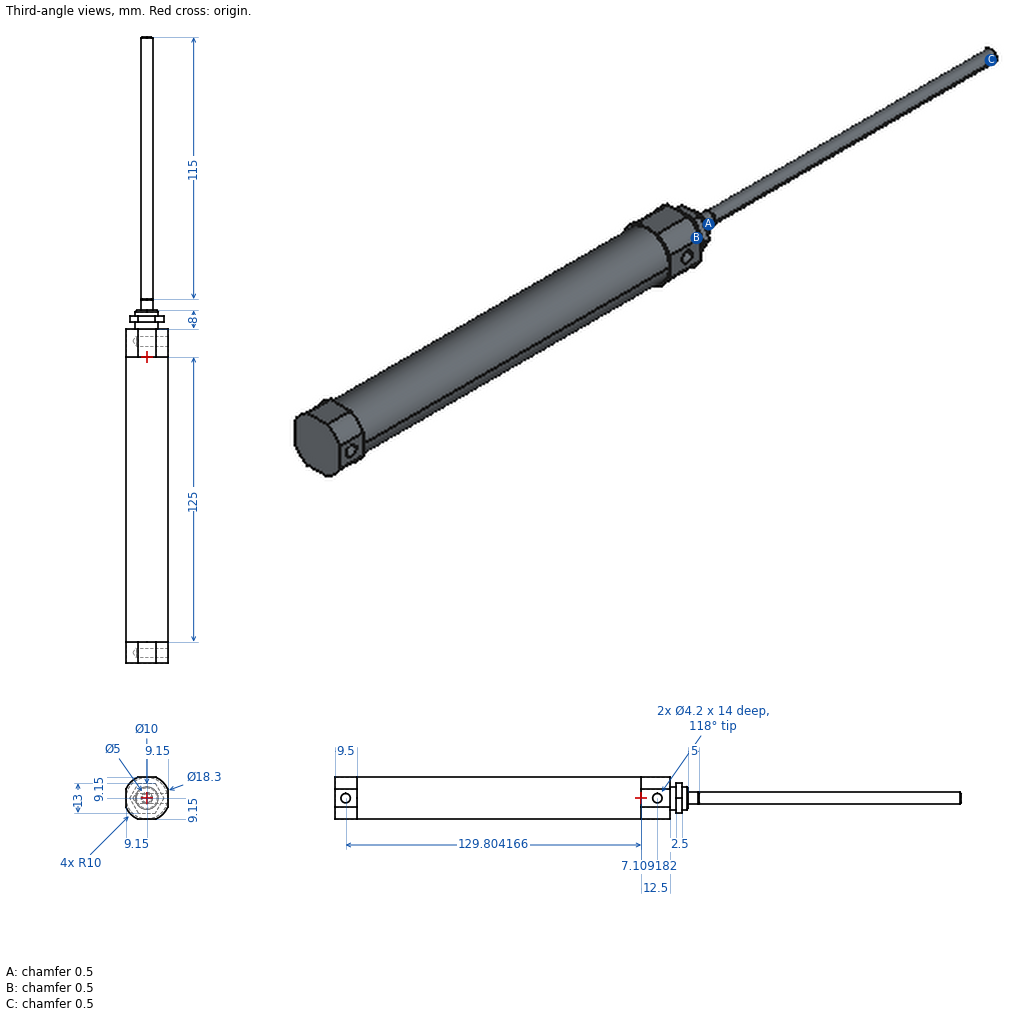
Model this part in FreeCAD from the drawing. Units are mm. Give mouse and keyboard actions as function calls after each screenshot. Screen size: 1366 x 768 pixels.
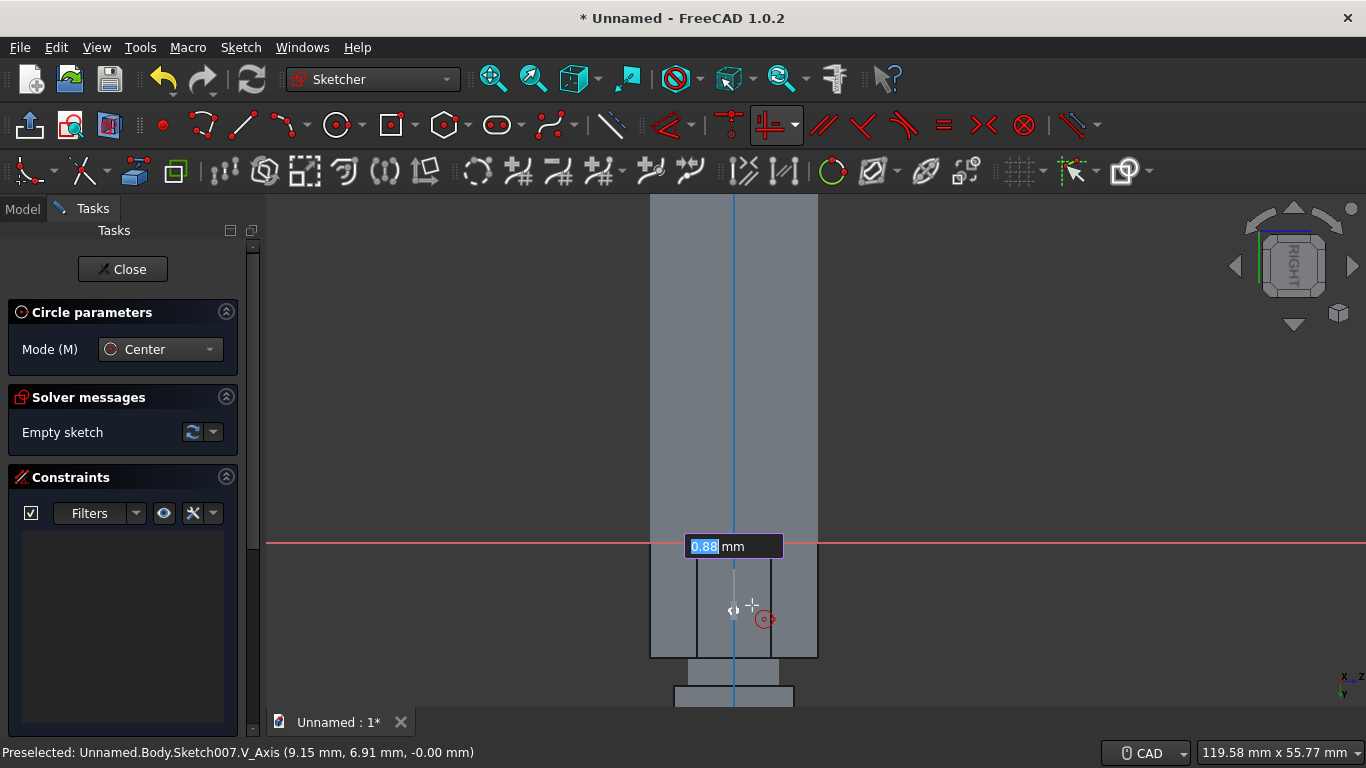
click(752, 602)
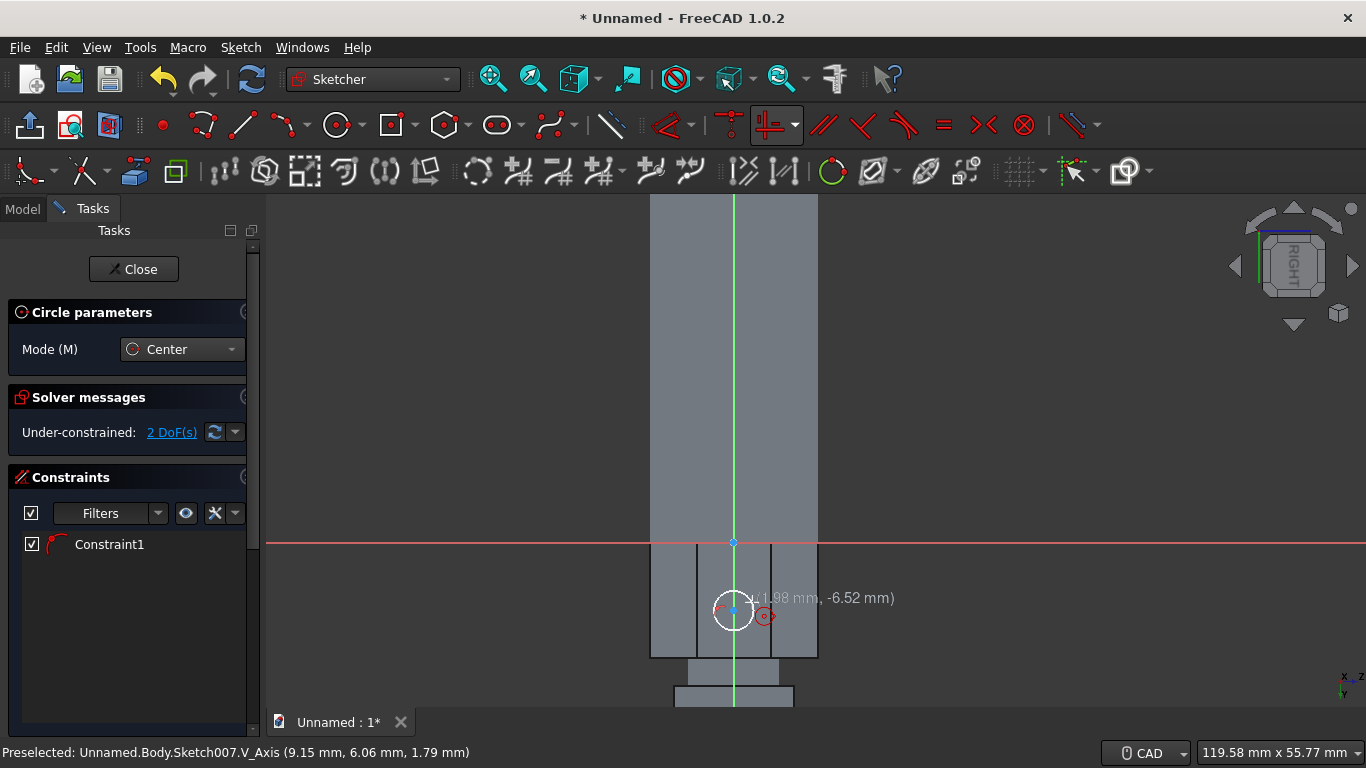
scroll(752, 605, down, 7)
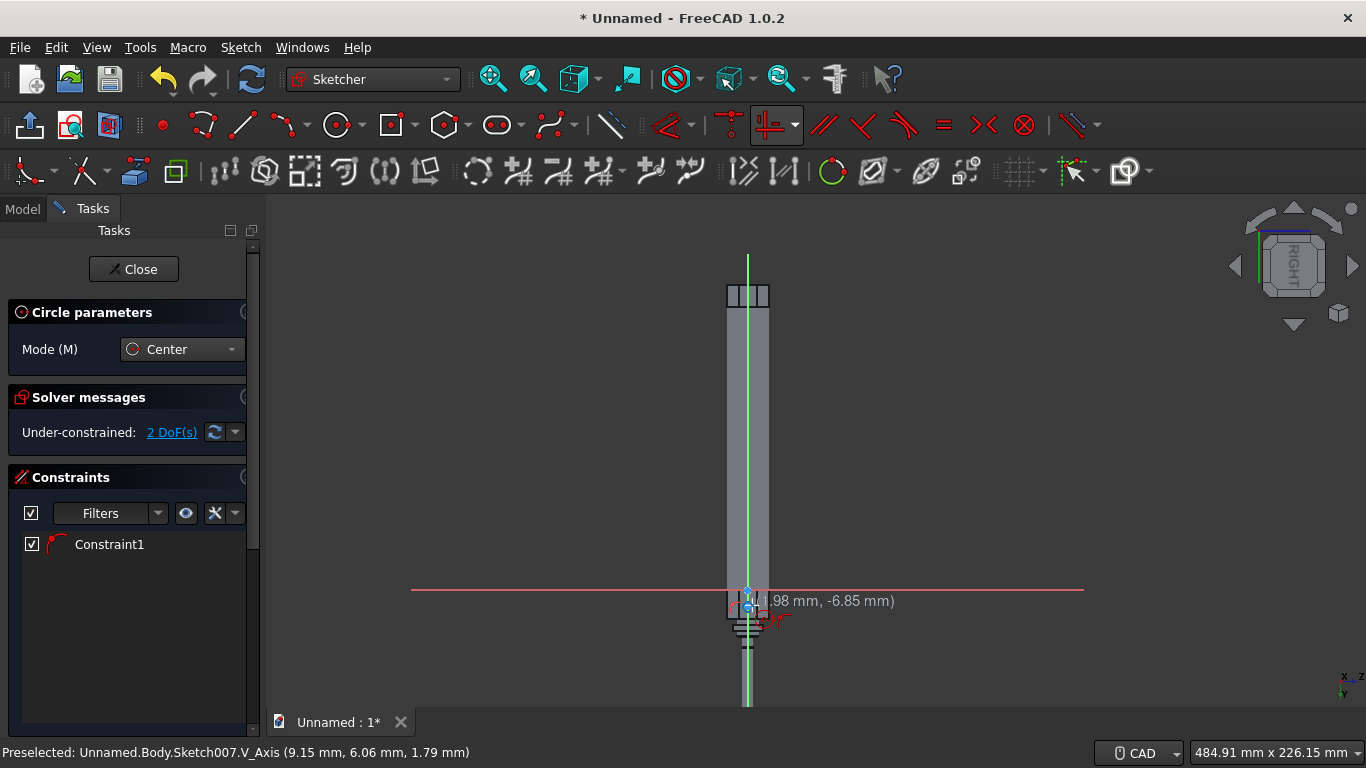
scroll(748, 296, up, 8)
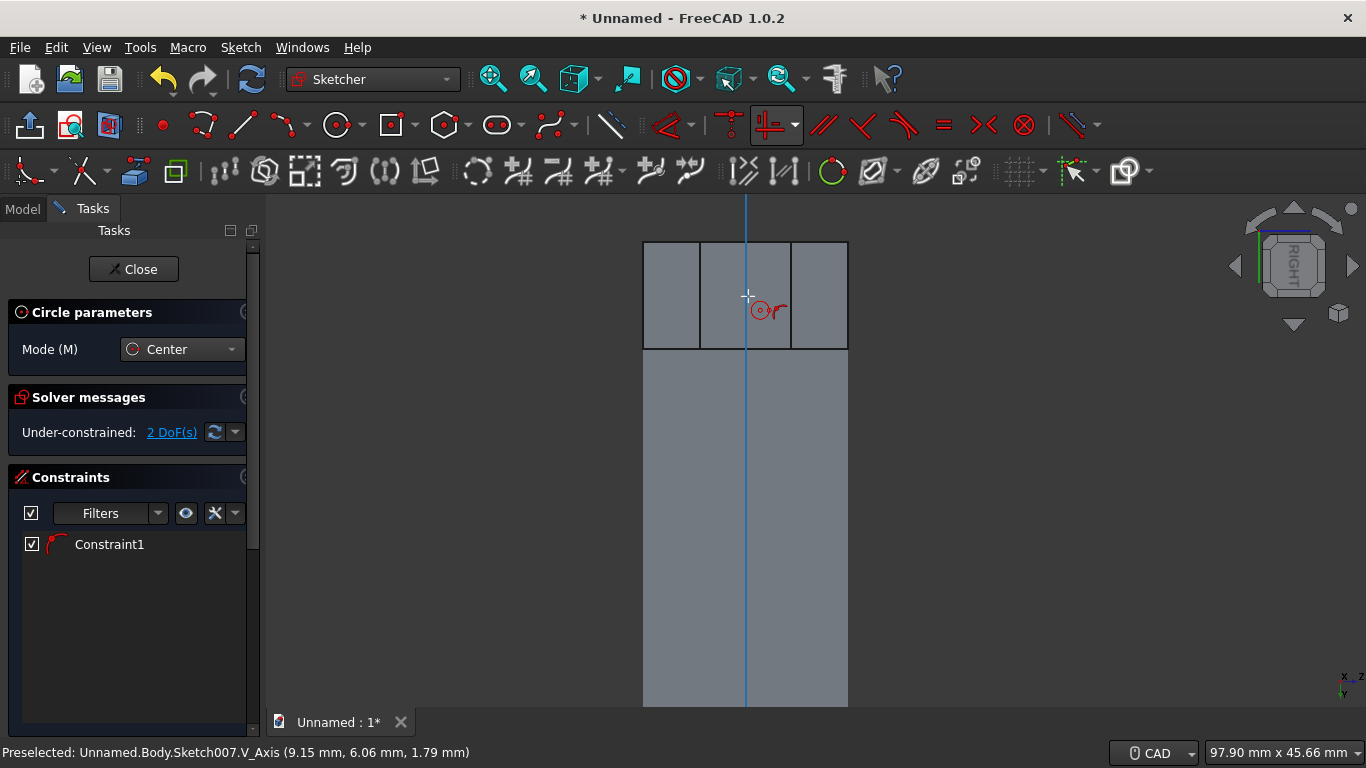
scroll(748, 295, down, 8)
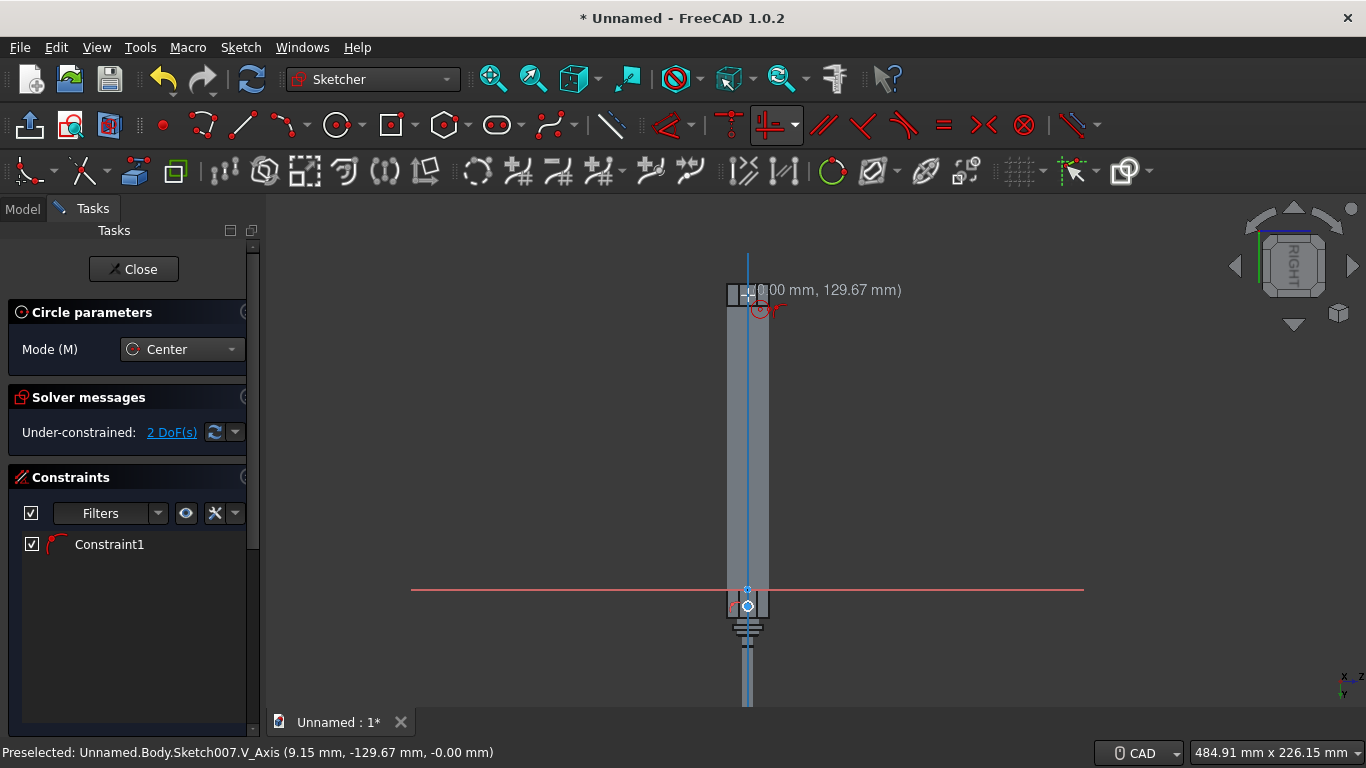
click(748, 295)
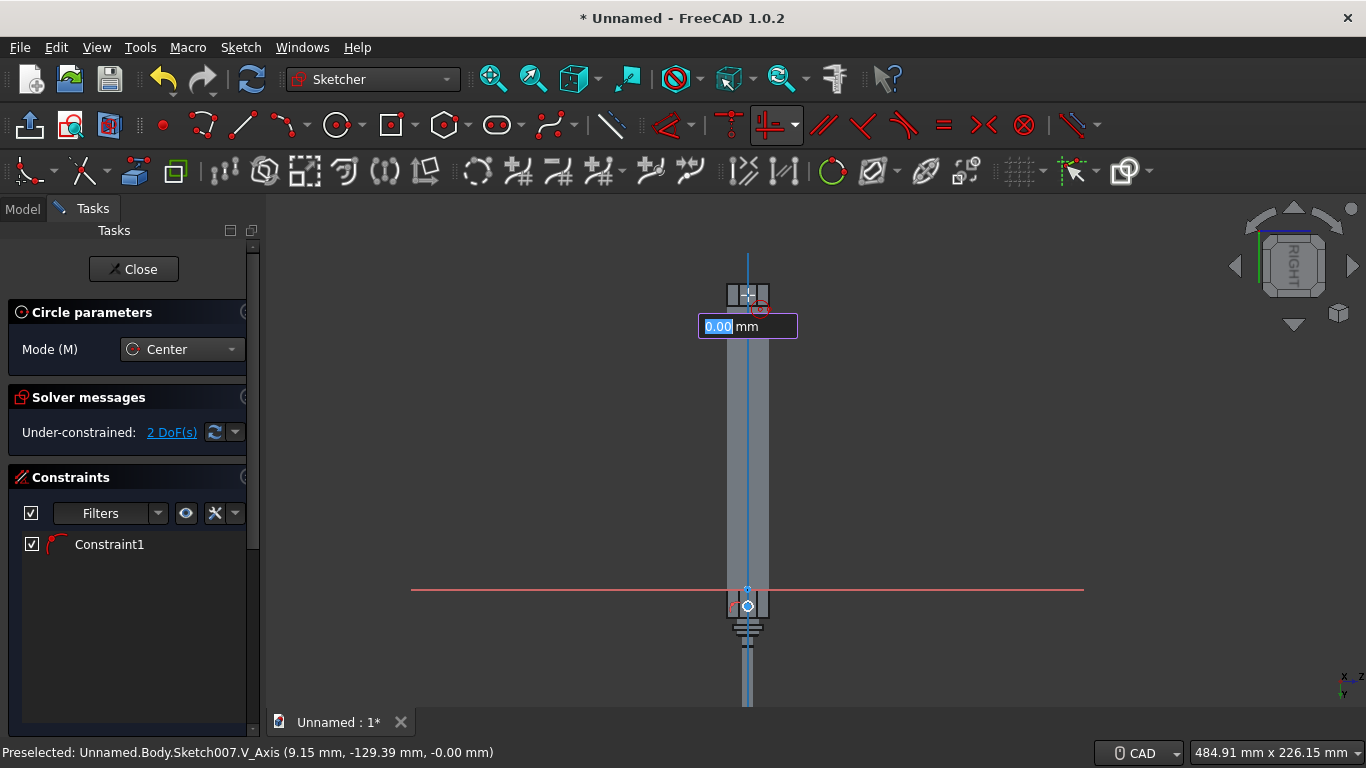
scroll(752, 293, up, 7)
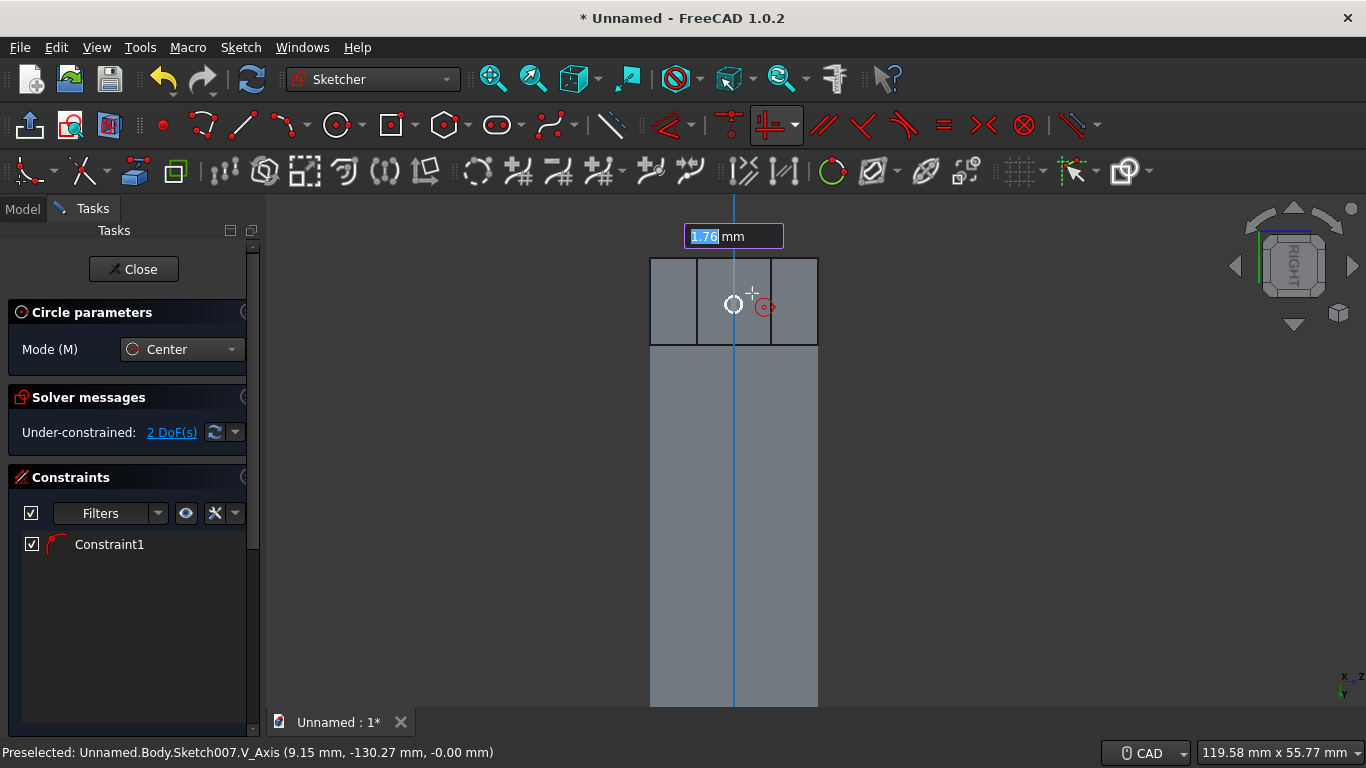
click(752, 294)
key(Escape)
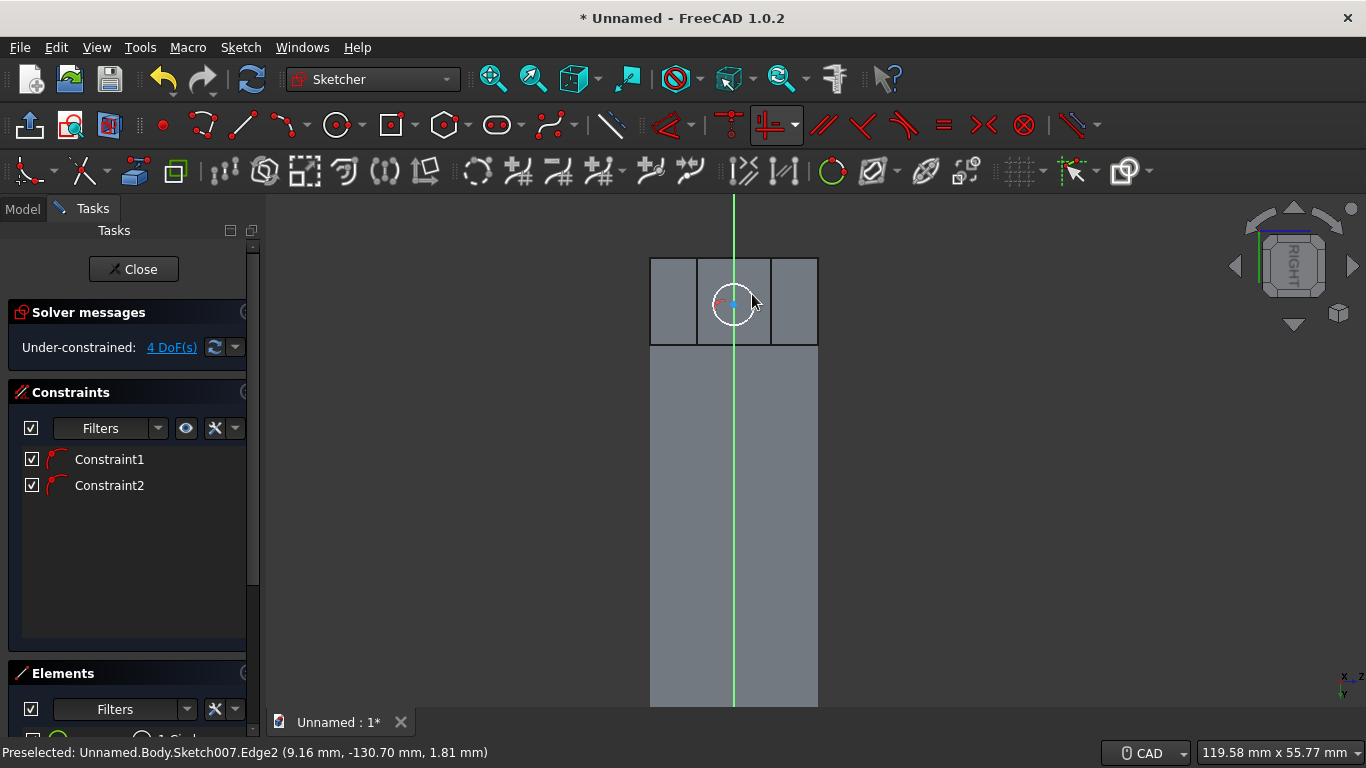
scroll(752, 293, down, 7)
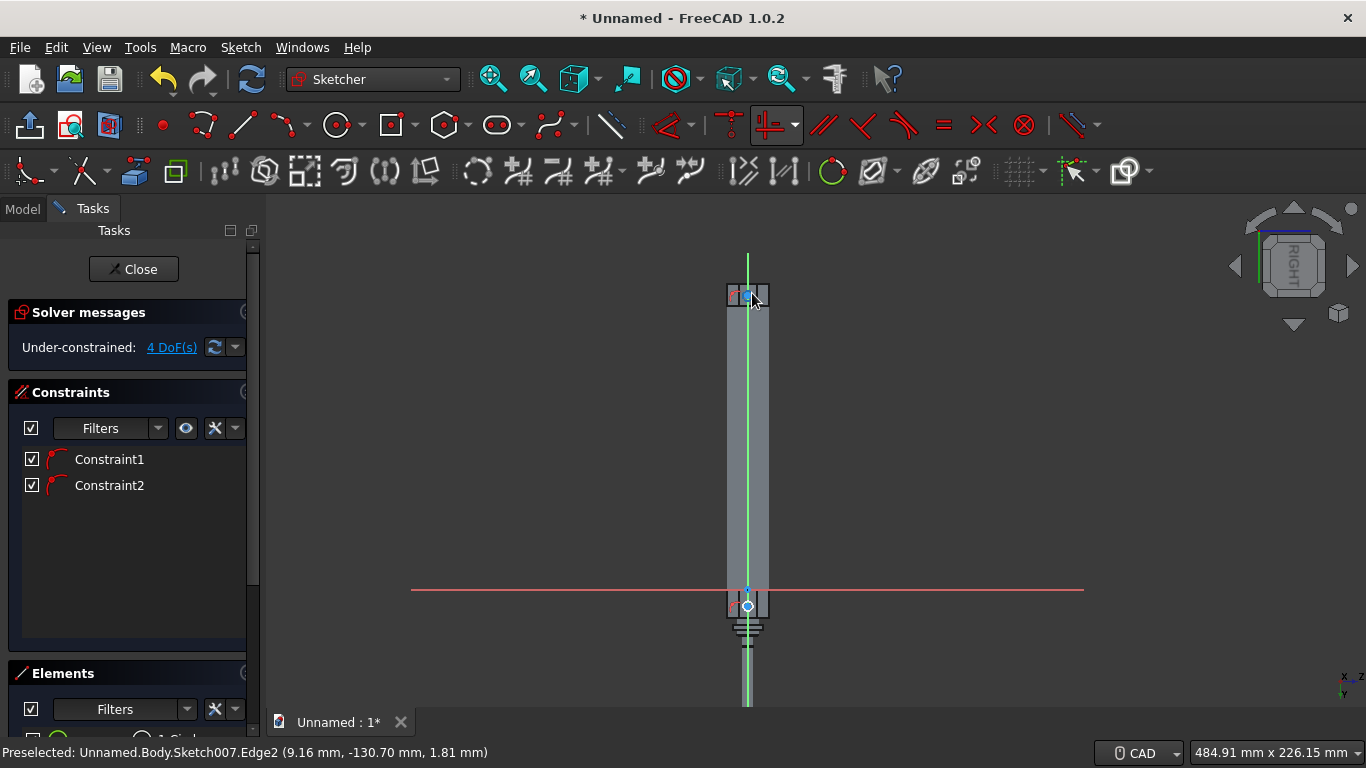
scroll(751, 603, up, 7)